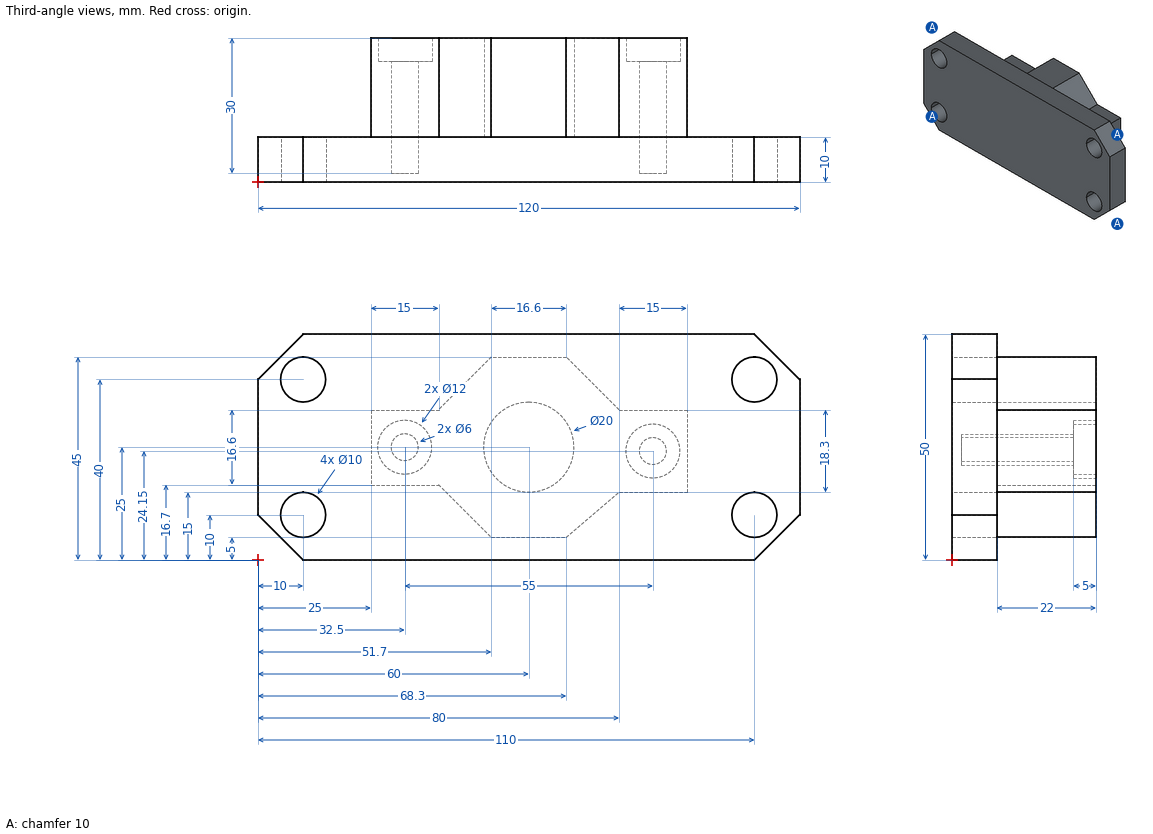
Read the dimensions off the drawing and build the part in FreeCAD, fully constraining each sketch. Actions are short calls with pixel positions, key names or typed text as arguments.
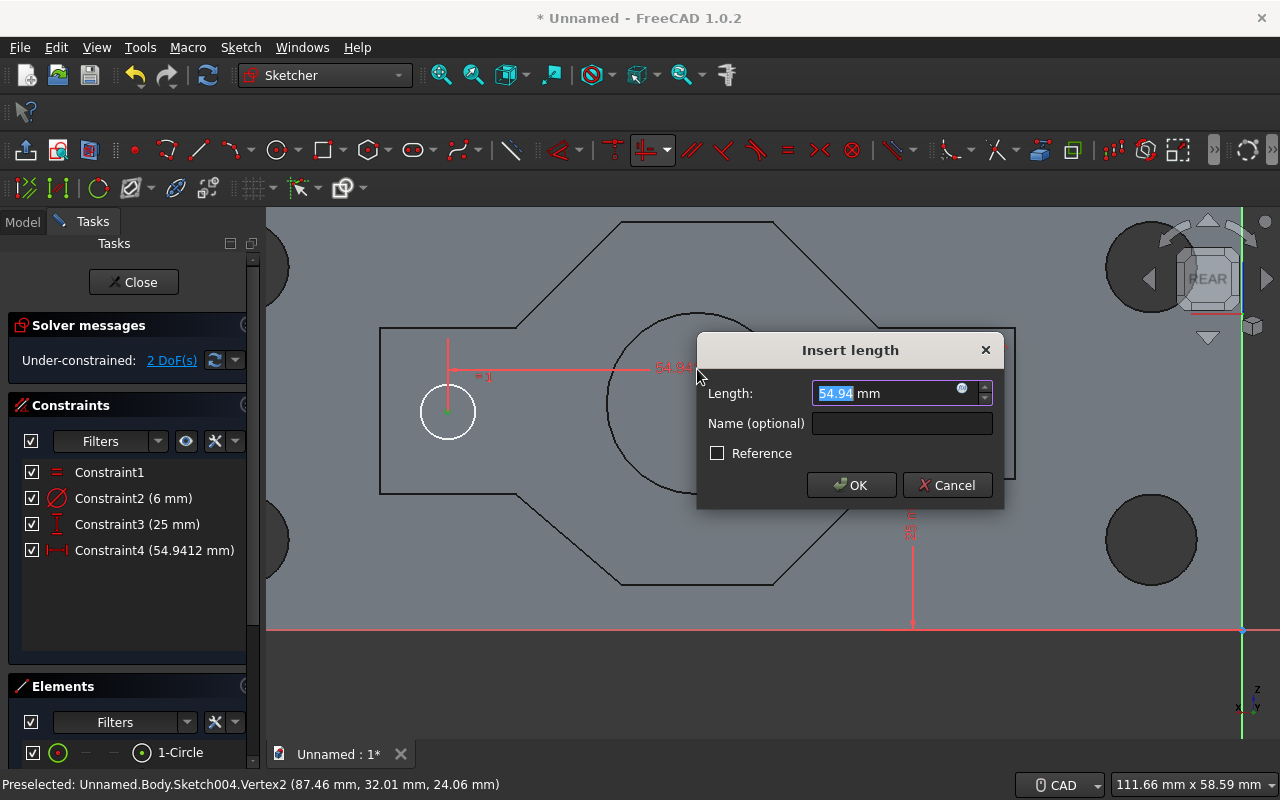
text(55)
key(Return)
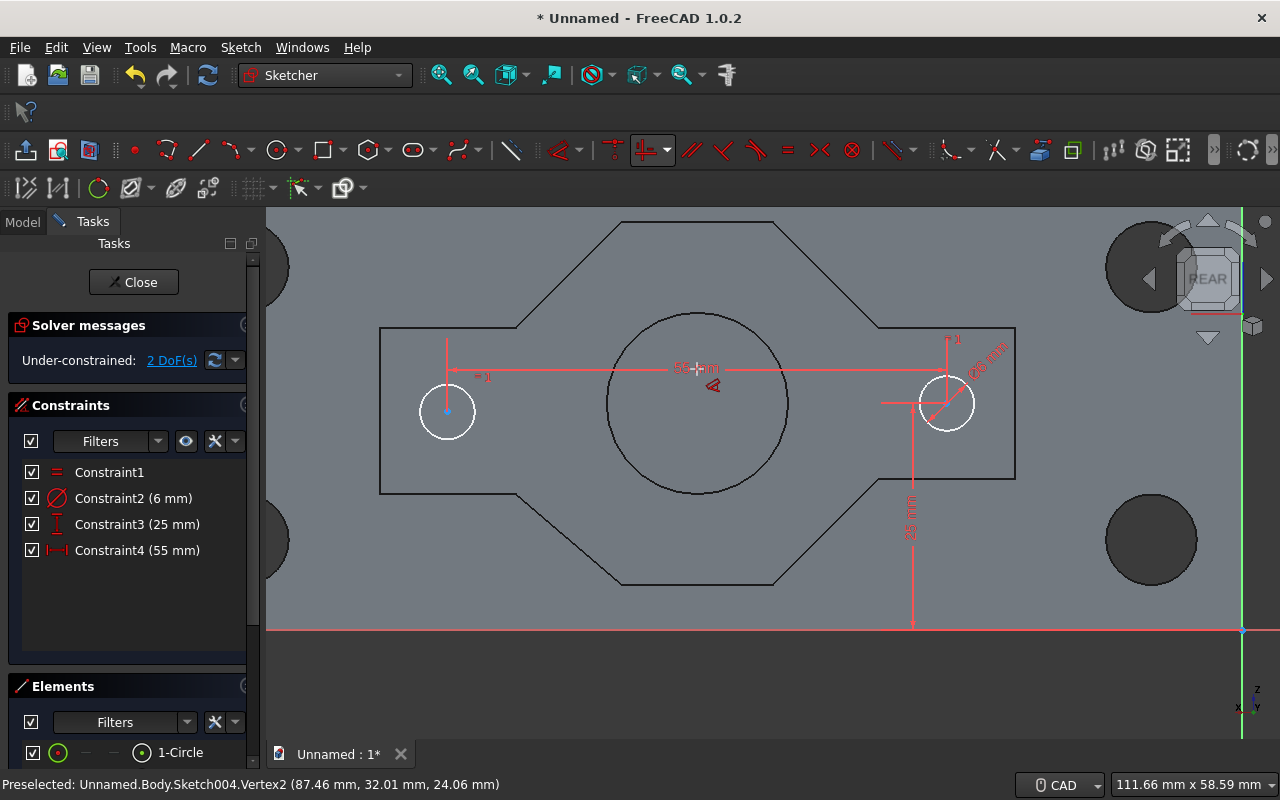
click(947, 403)
click(1031, 664)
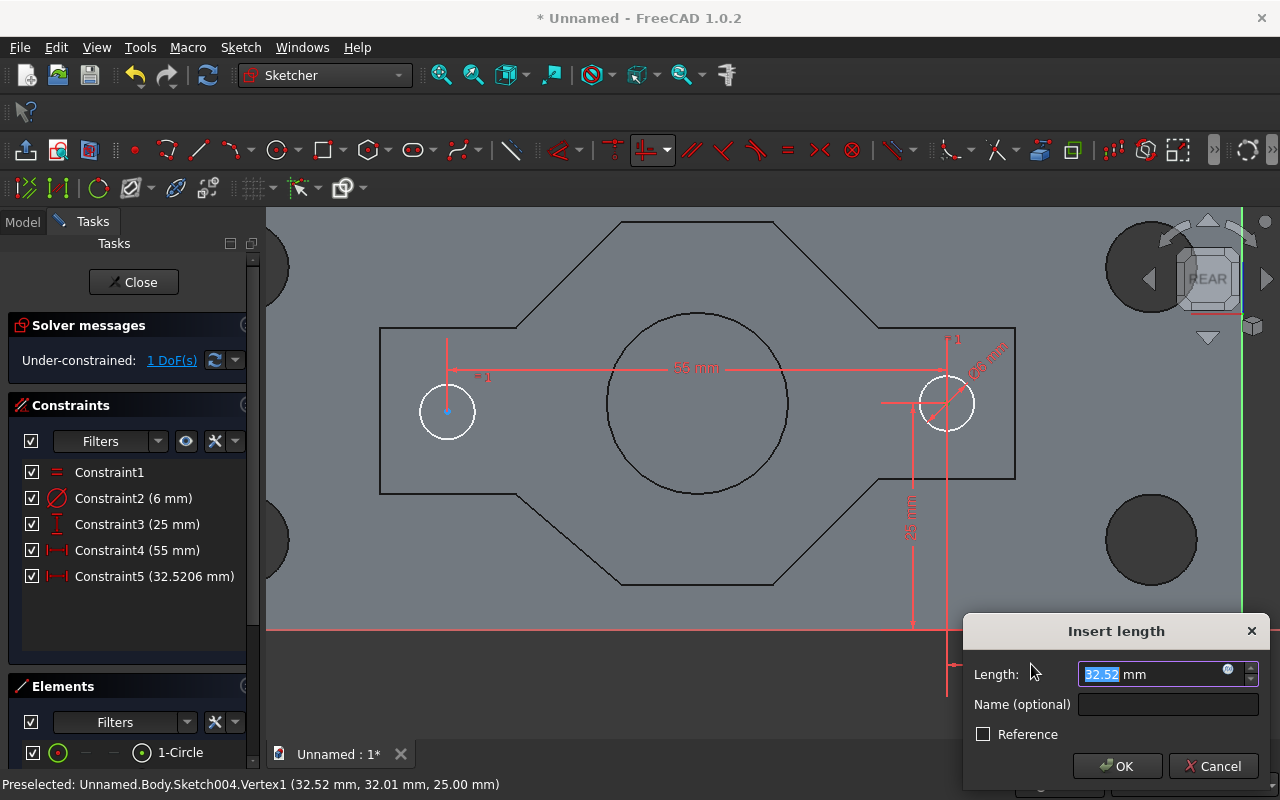
text(32.5)
key(Return)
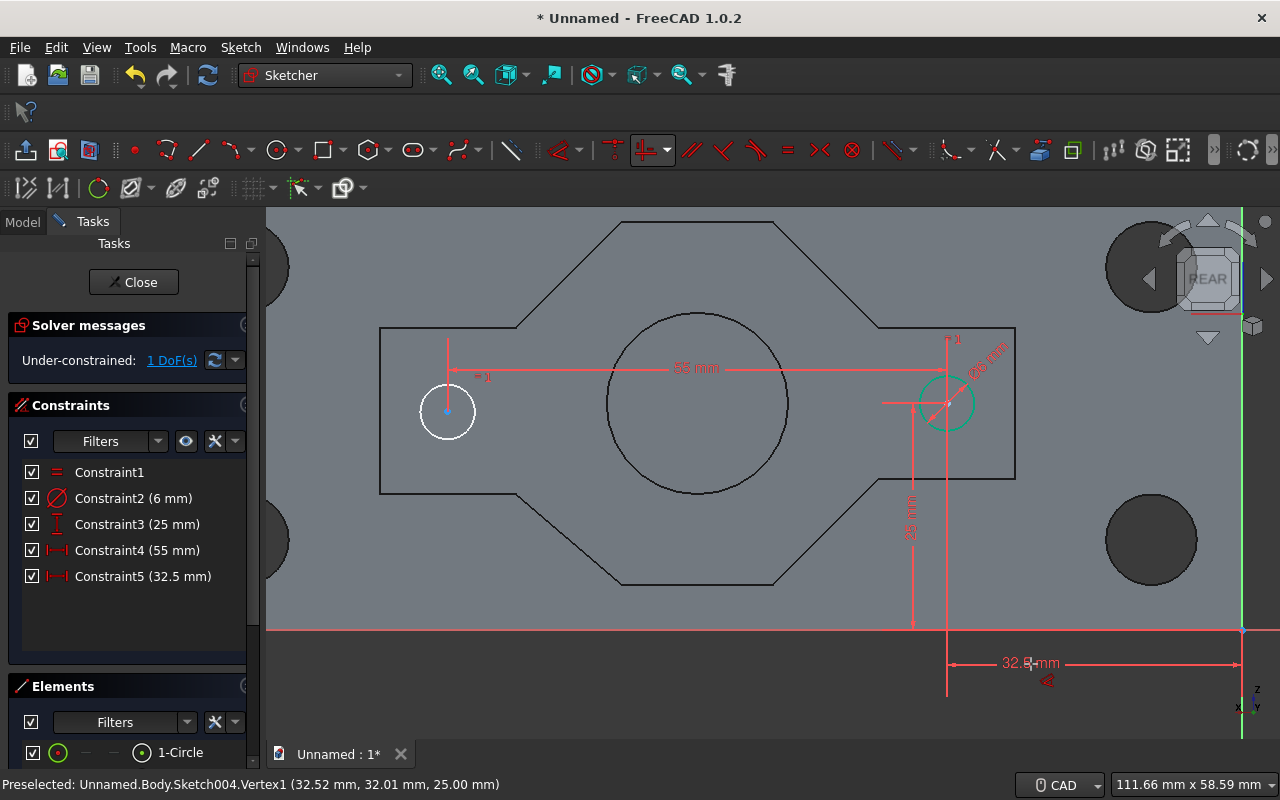
click(448, 412)
click(414, 521)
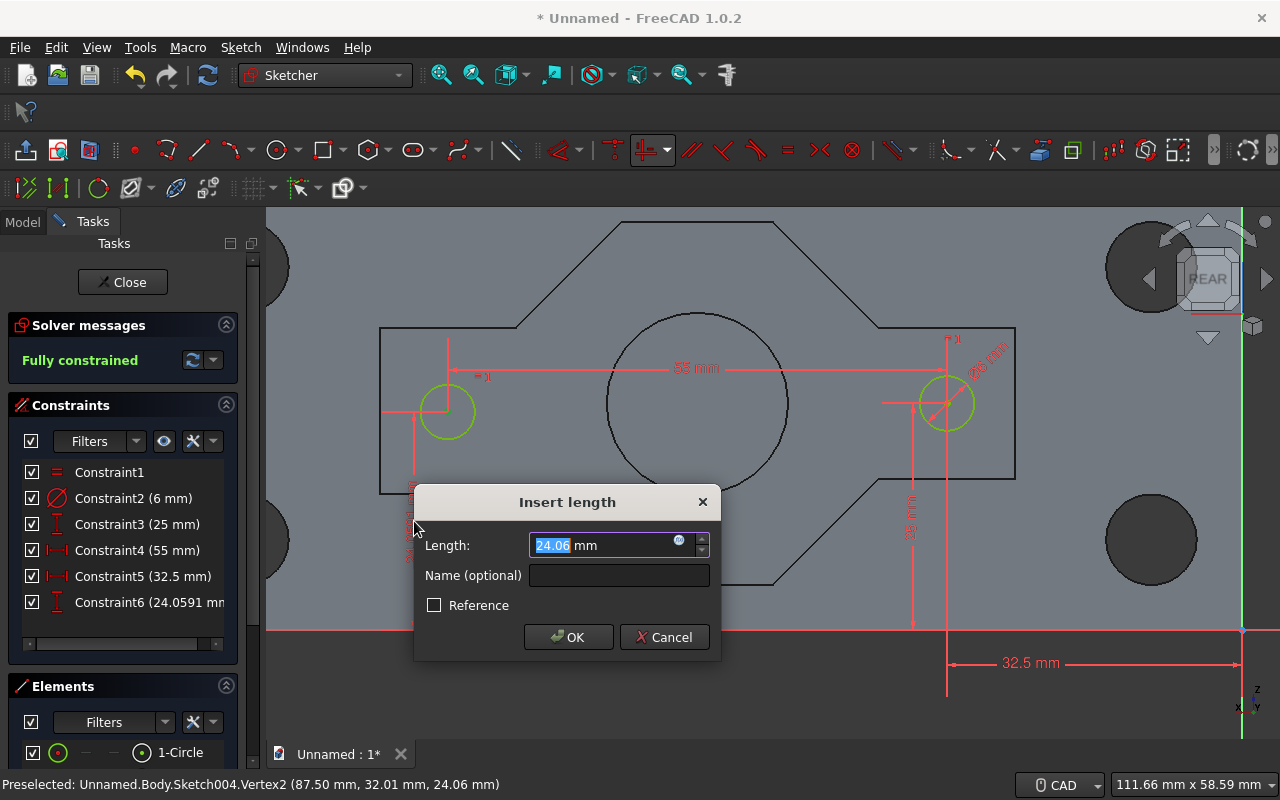
text(24.15)
key(Return)
key(Escape)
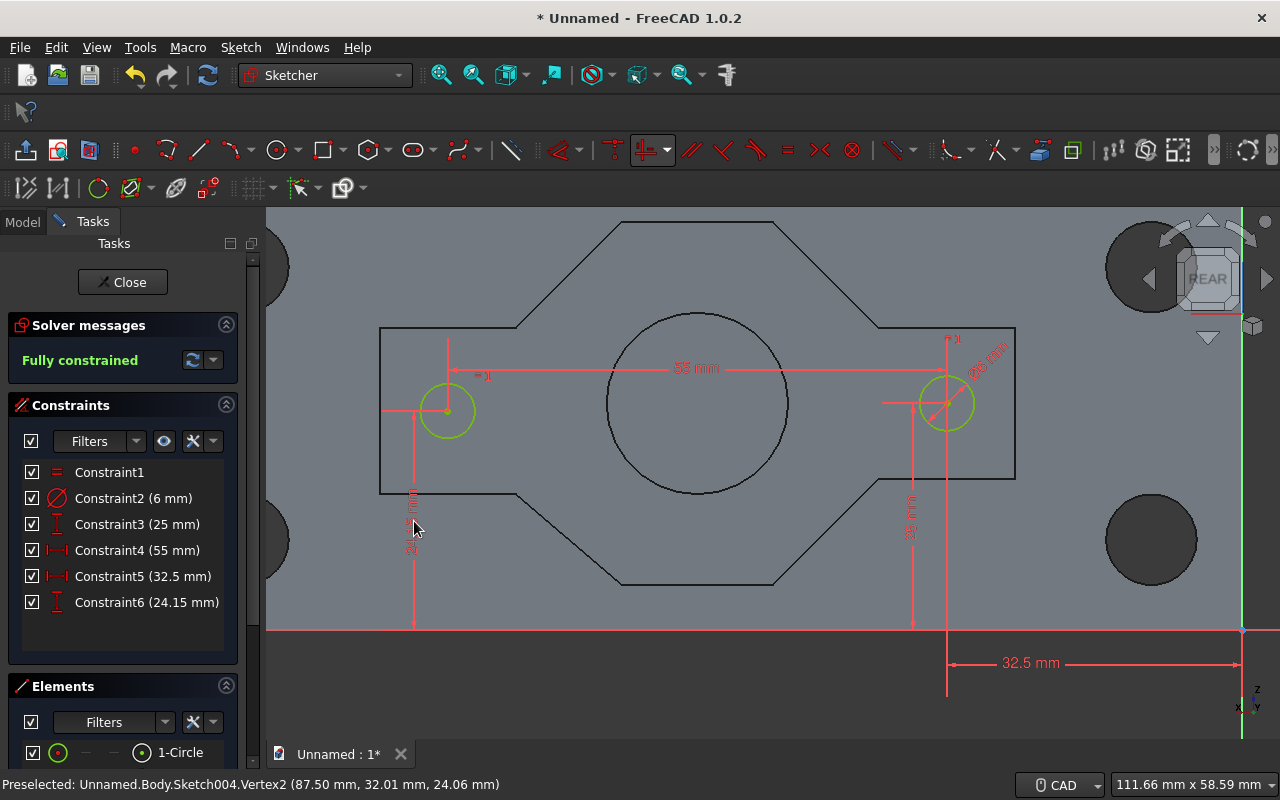
click(123, 282)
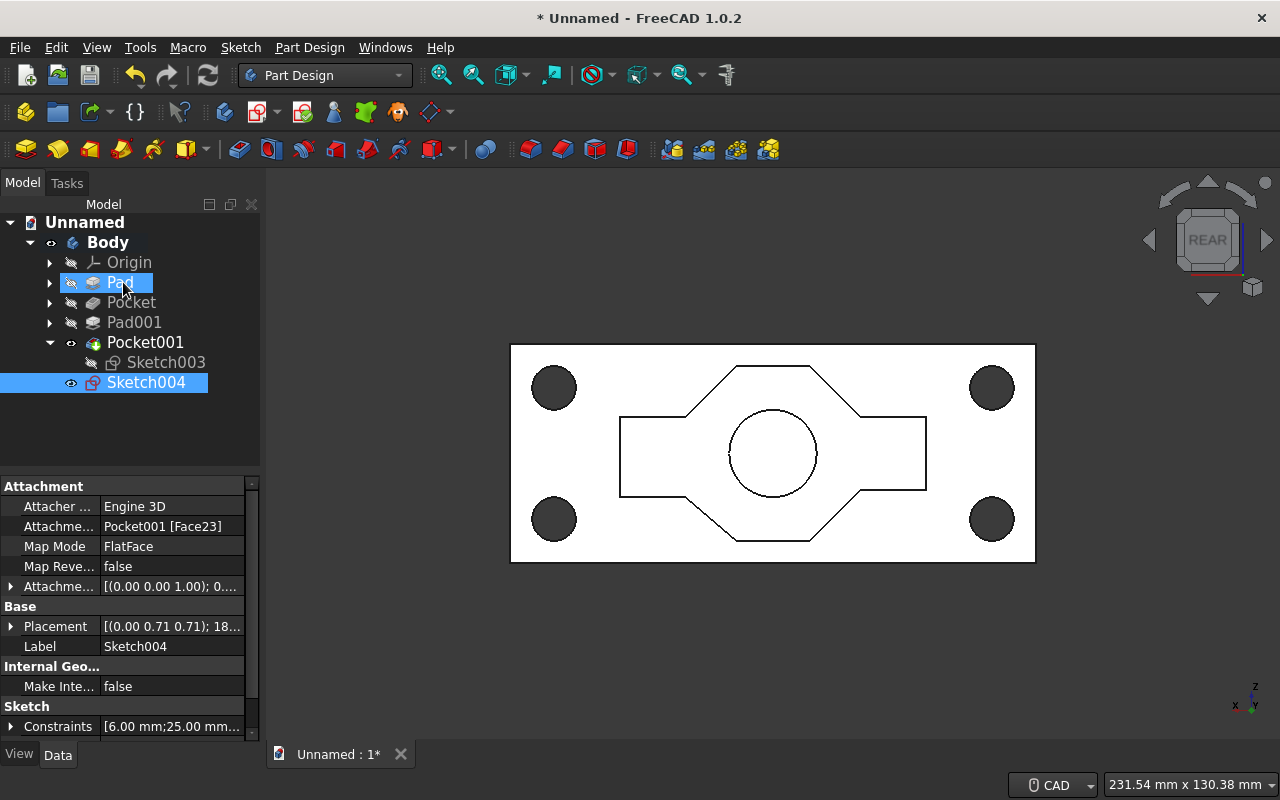
click(240, 150)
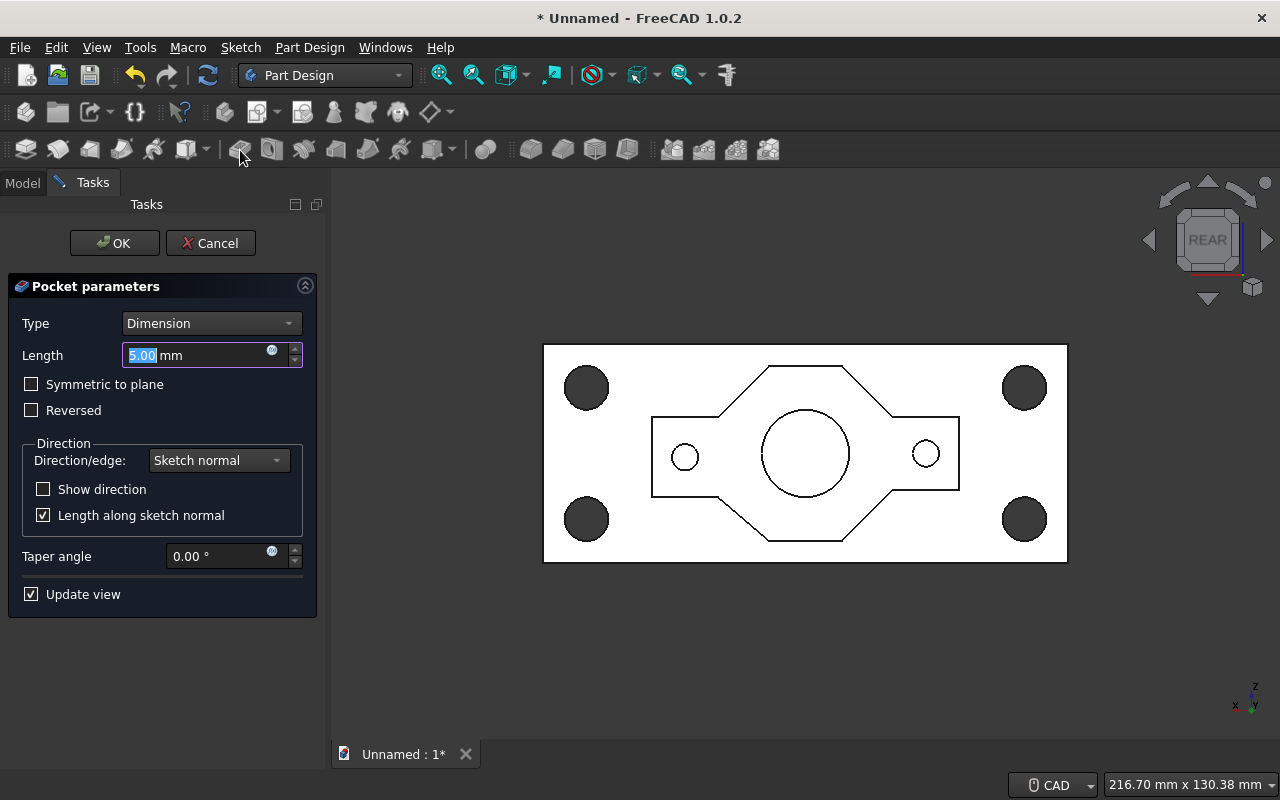
text(30)
key(Tab)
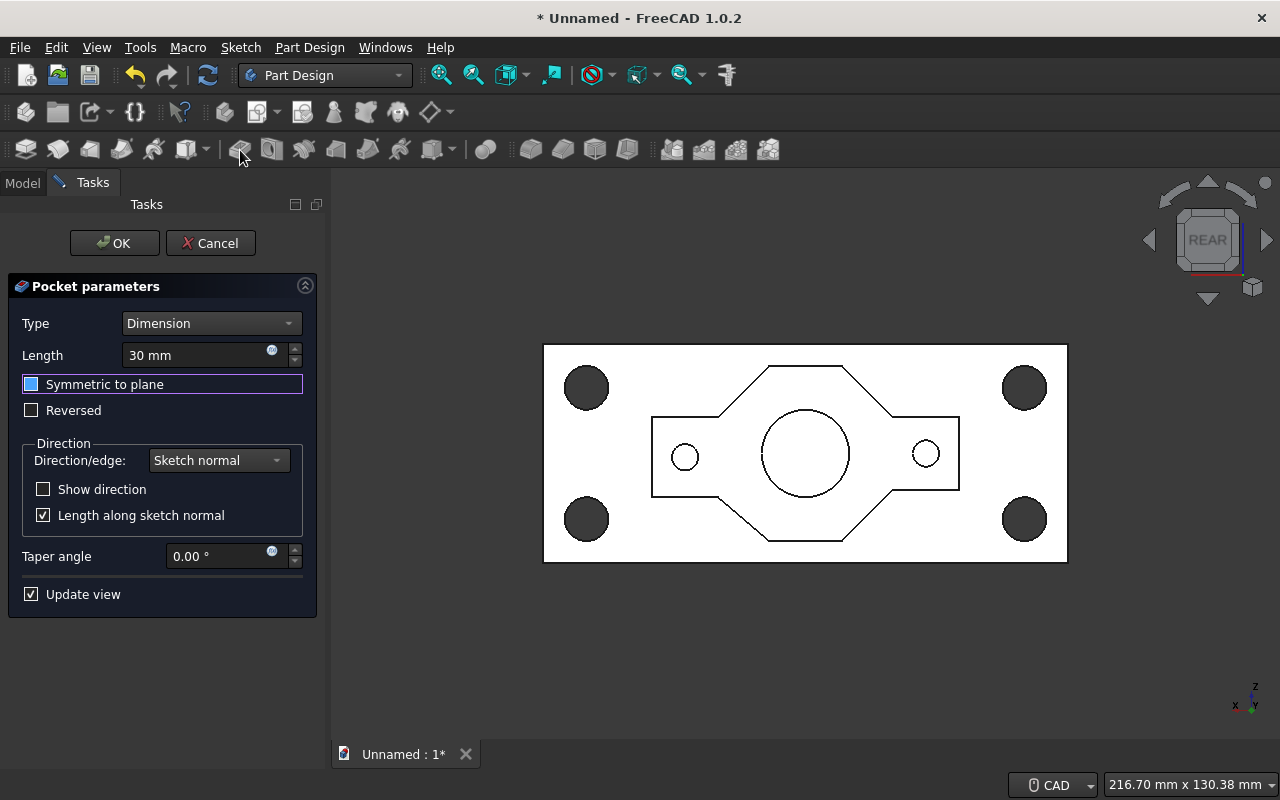
click(115, 243)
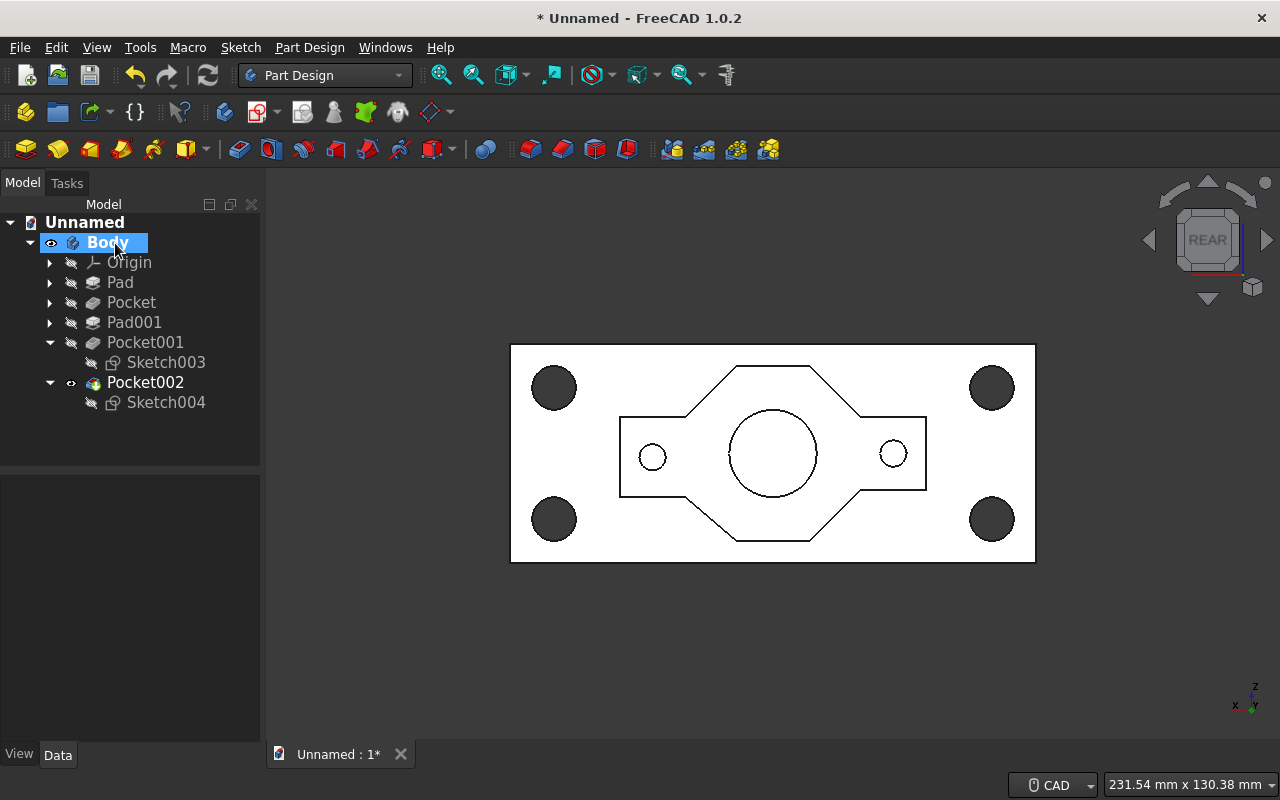
click(729, 503)